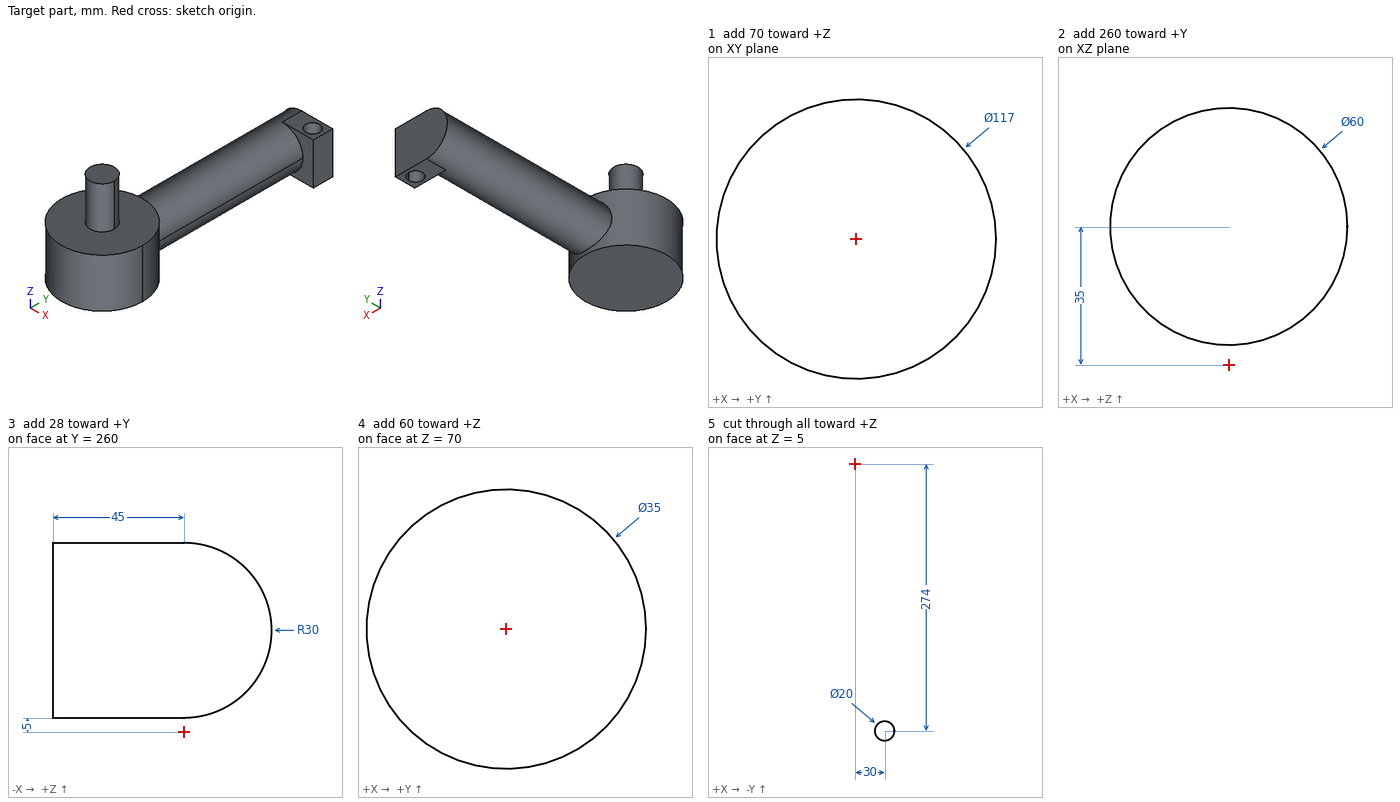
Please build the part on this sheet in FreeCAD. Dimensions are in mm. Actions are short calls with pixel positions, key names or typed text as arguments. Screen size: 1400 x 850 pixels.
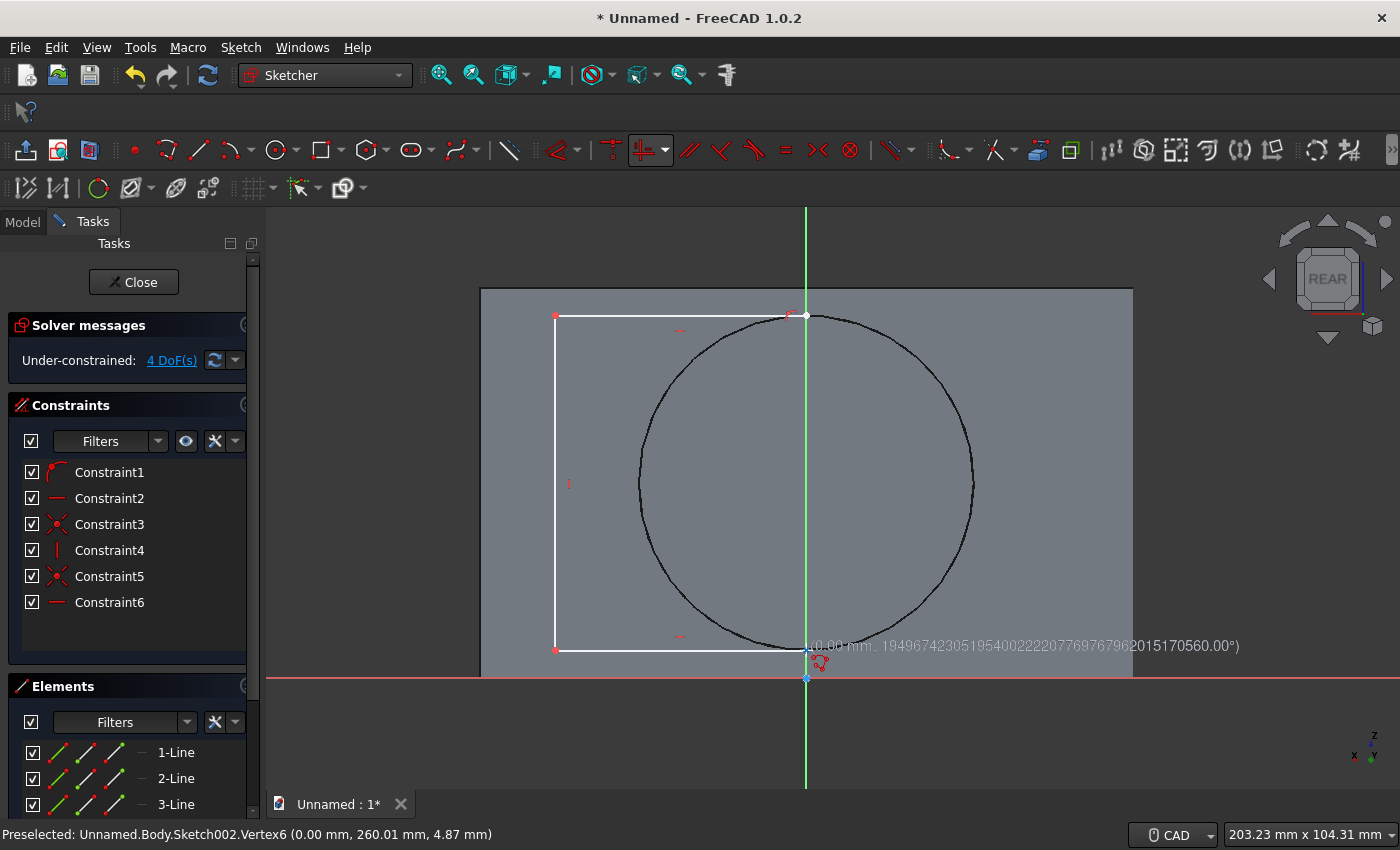
key(g)
key(3)
key(a)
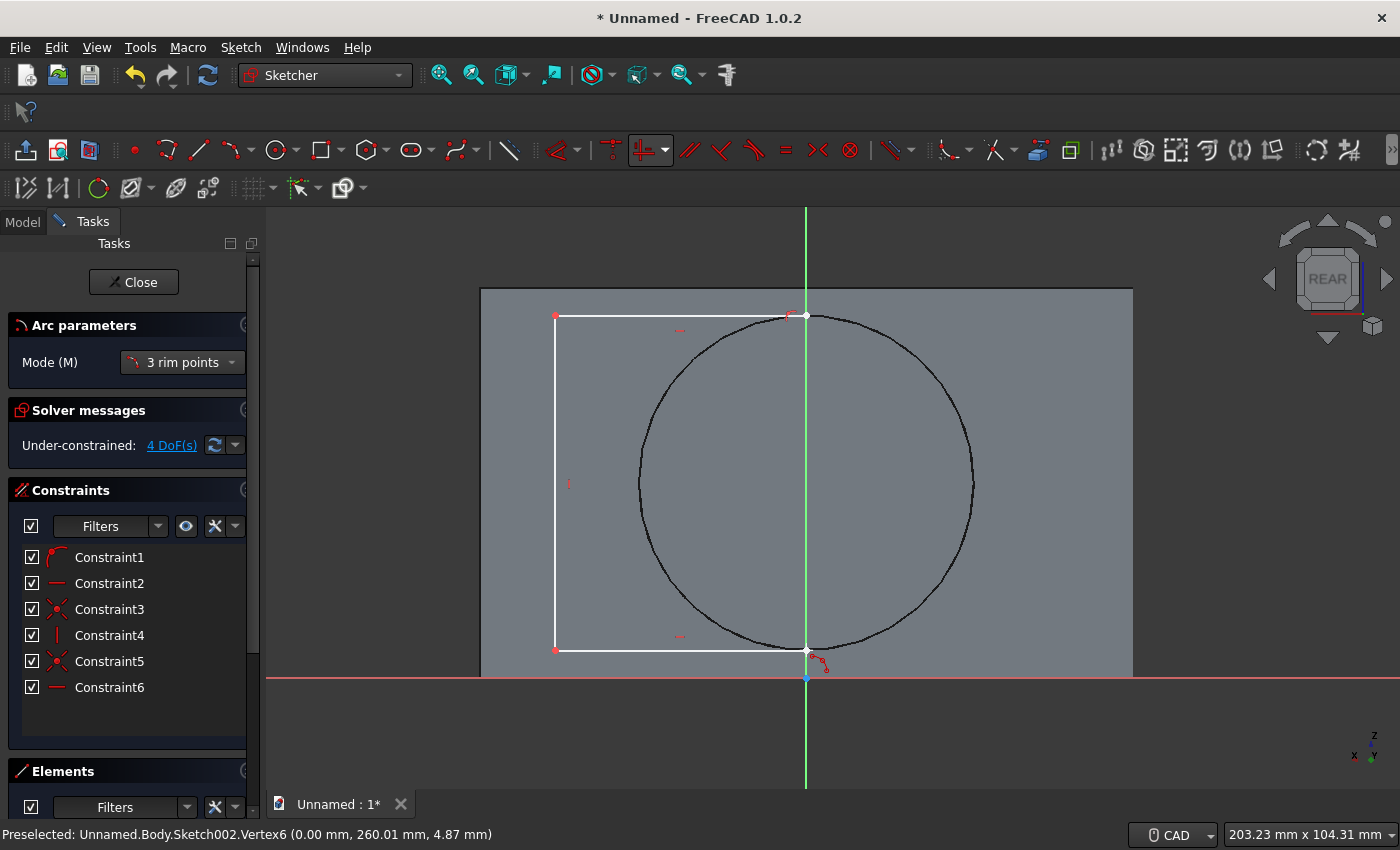
click(806, 651)
click(806, 316)
click(974, 483)
key(Escape)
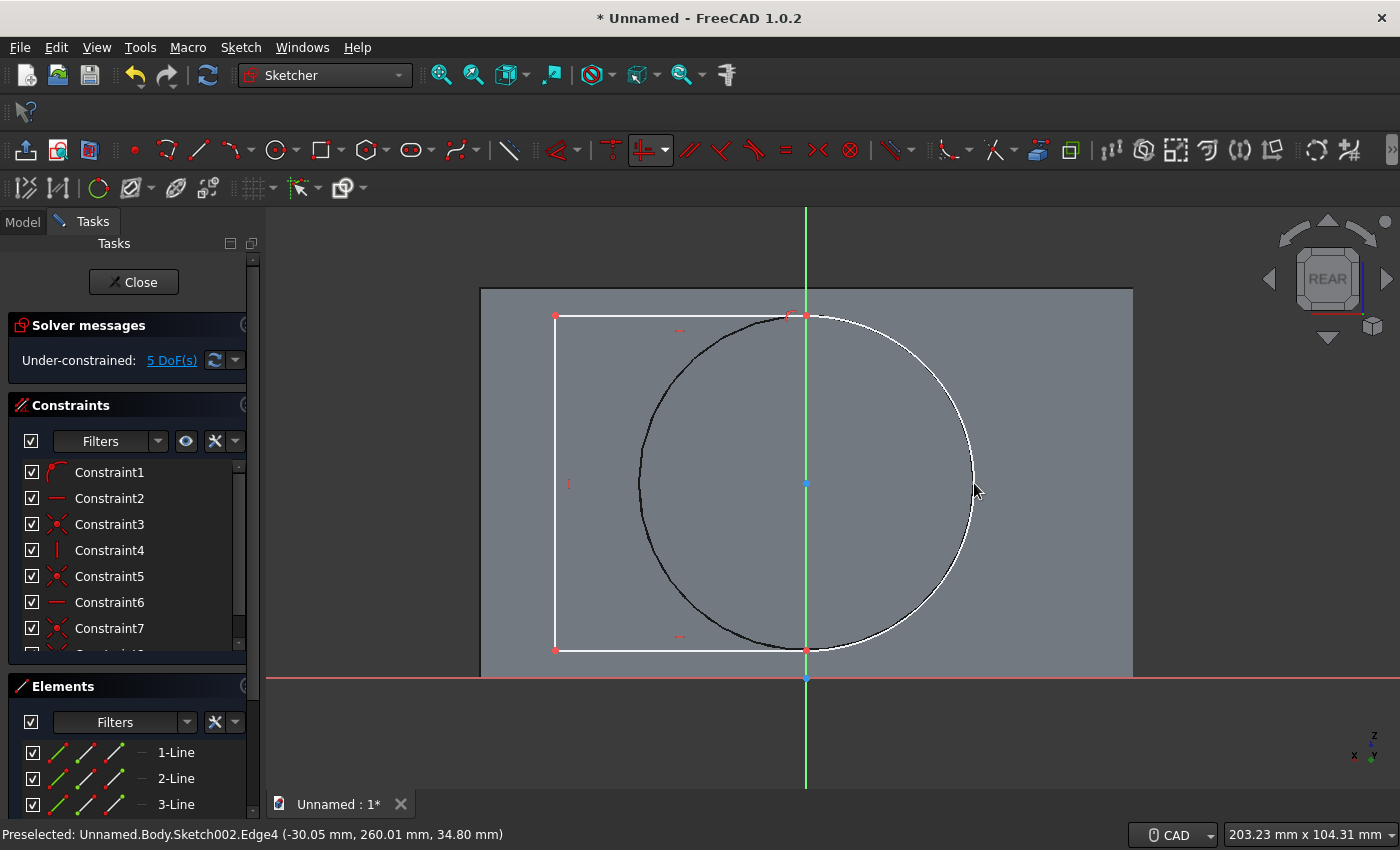
click(731, 316)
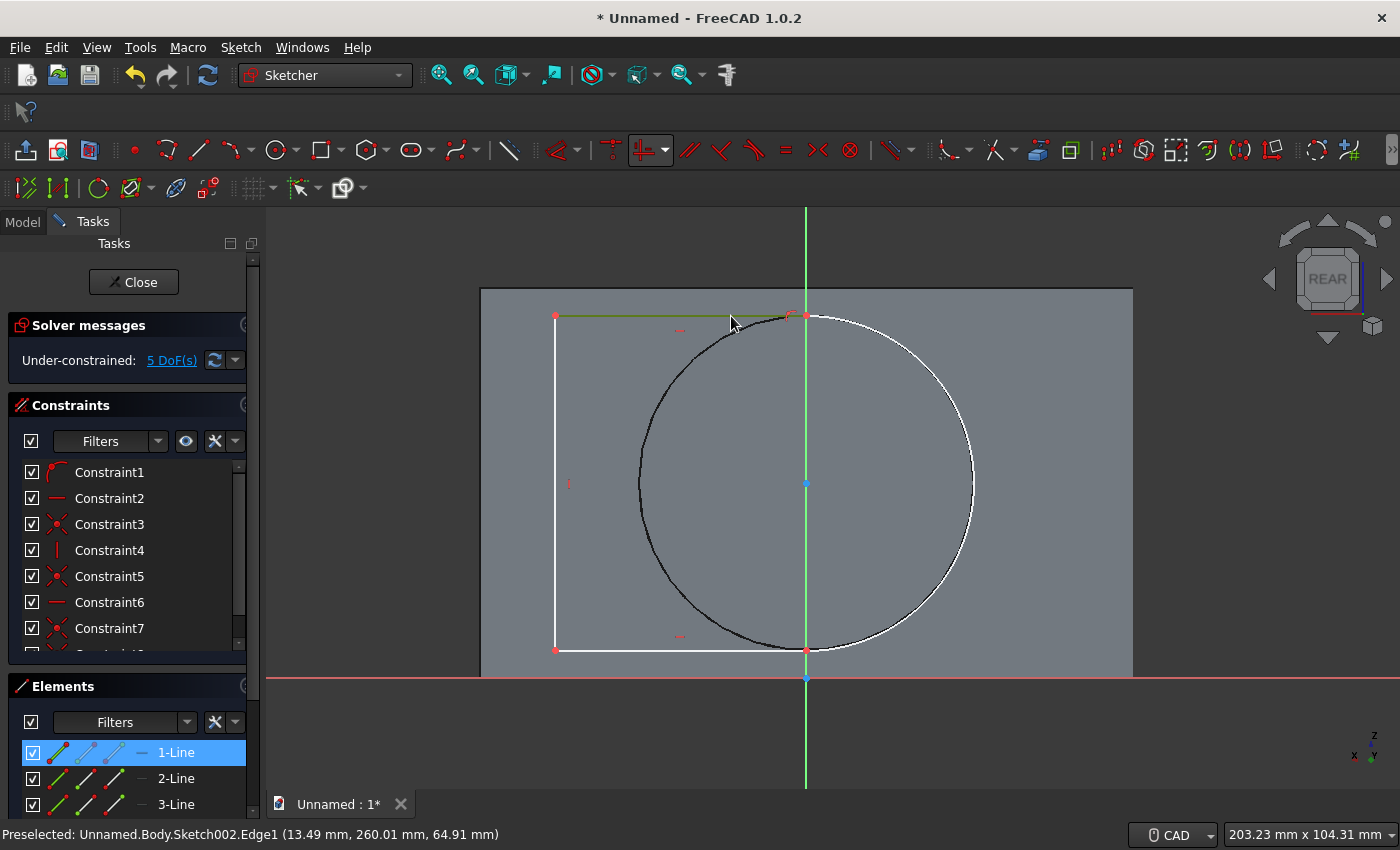
click(942, 582)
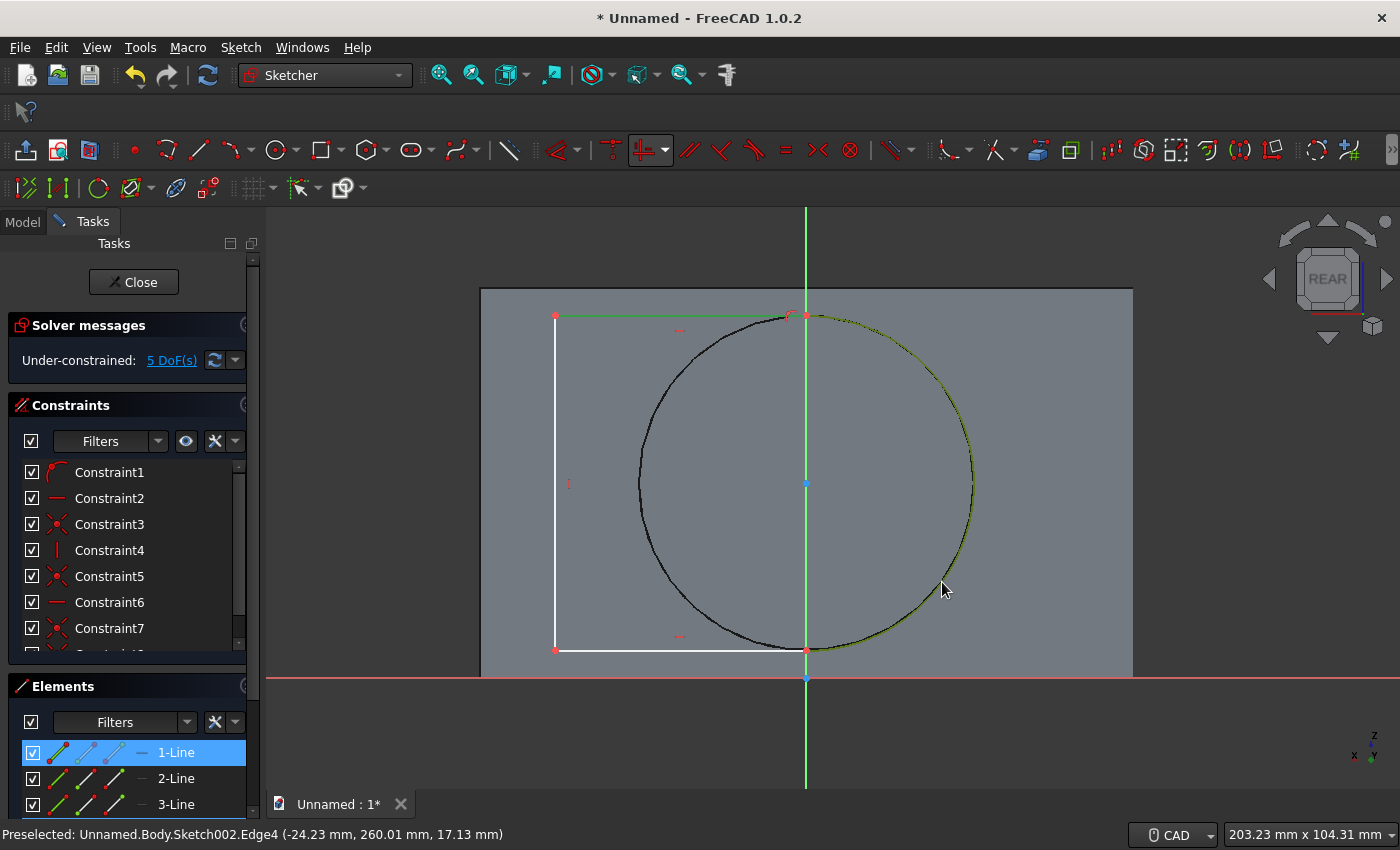
key(t)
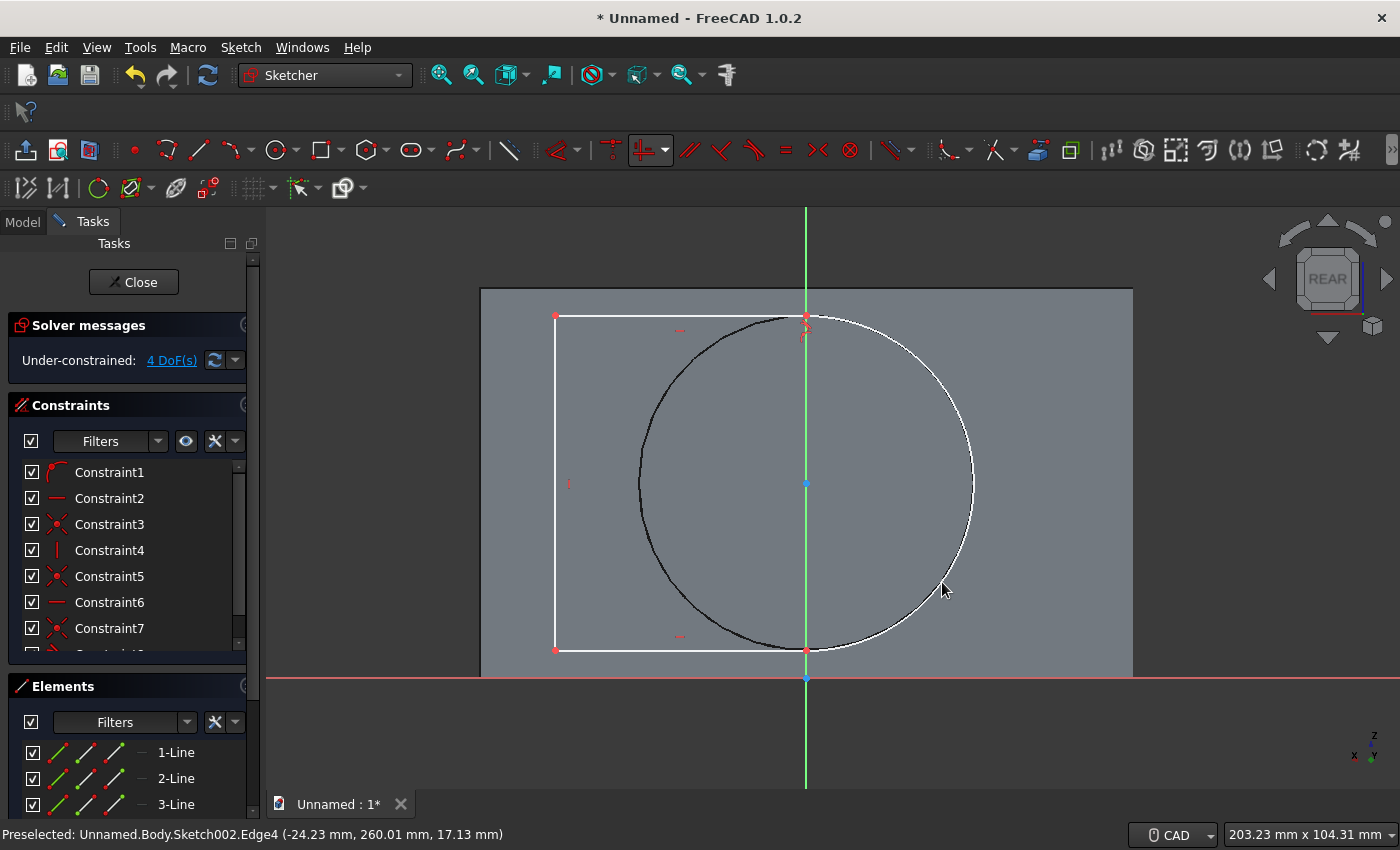
click(630, 651)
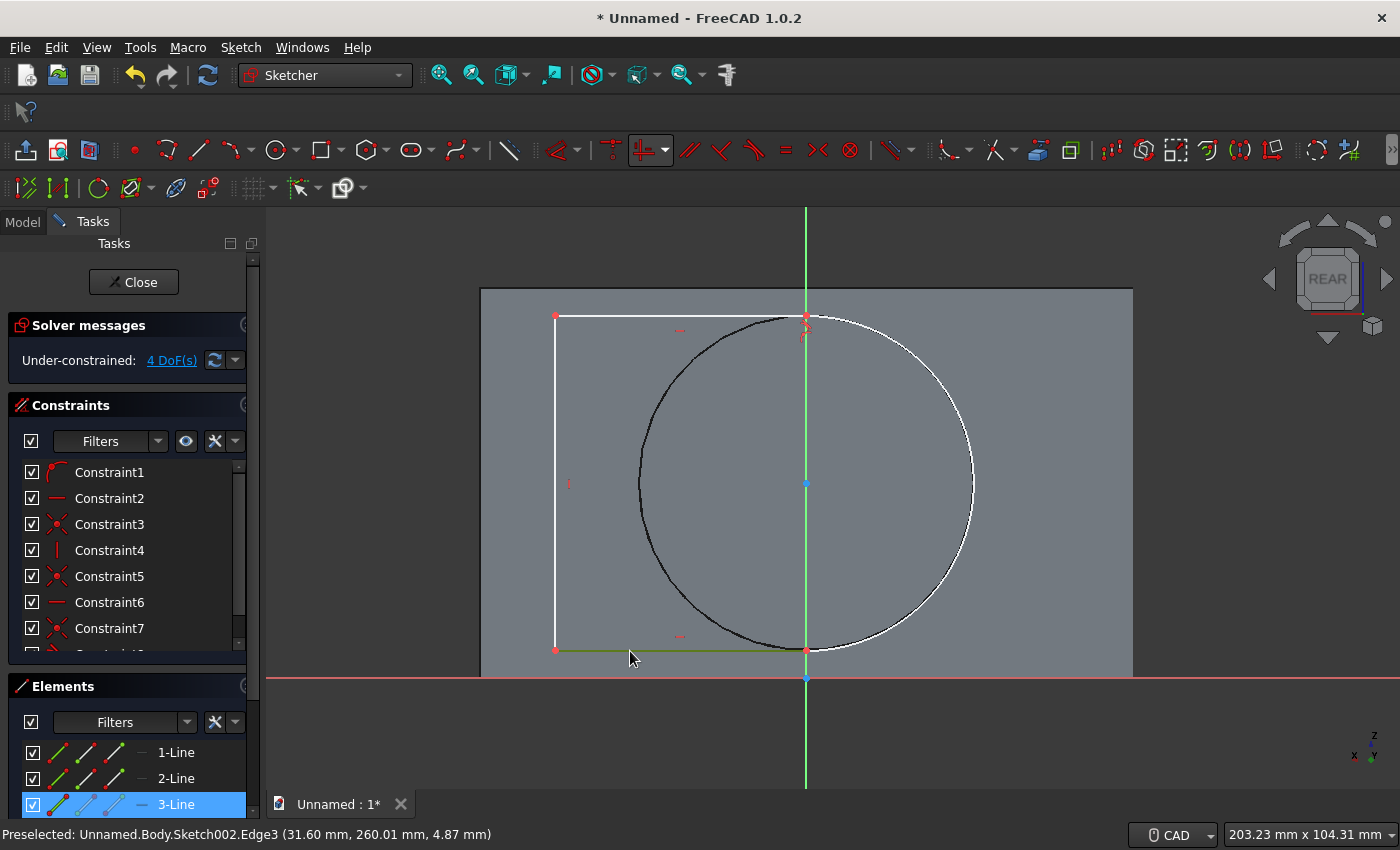
click(942, 582)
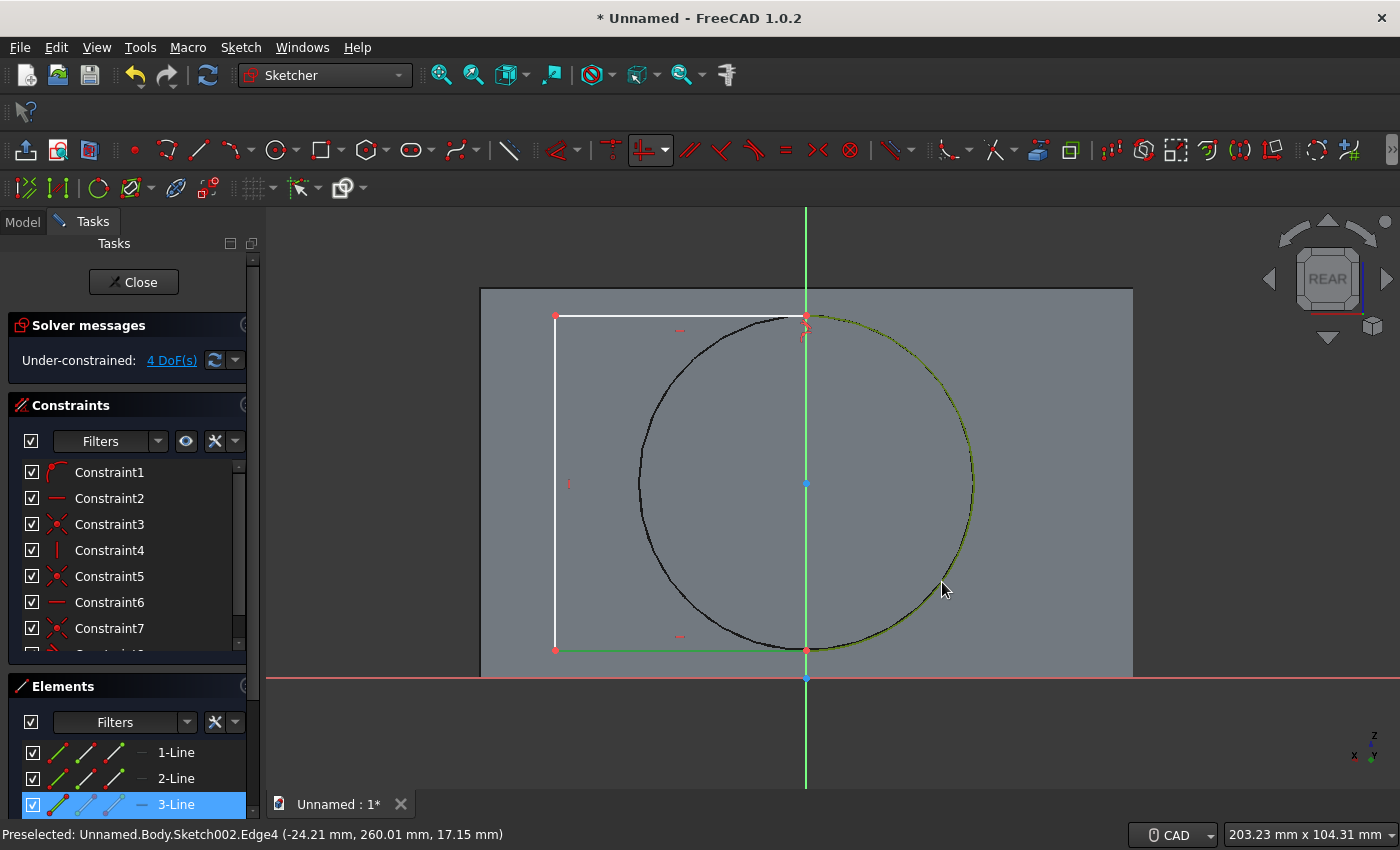
click(754, 150)